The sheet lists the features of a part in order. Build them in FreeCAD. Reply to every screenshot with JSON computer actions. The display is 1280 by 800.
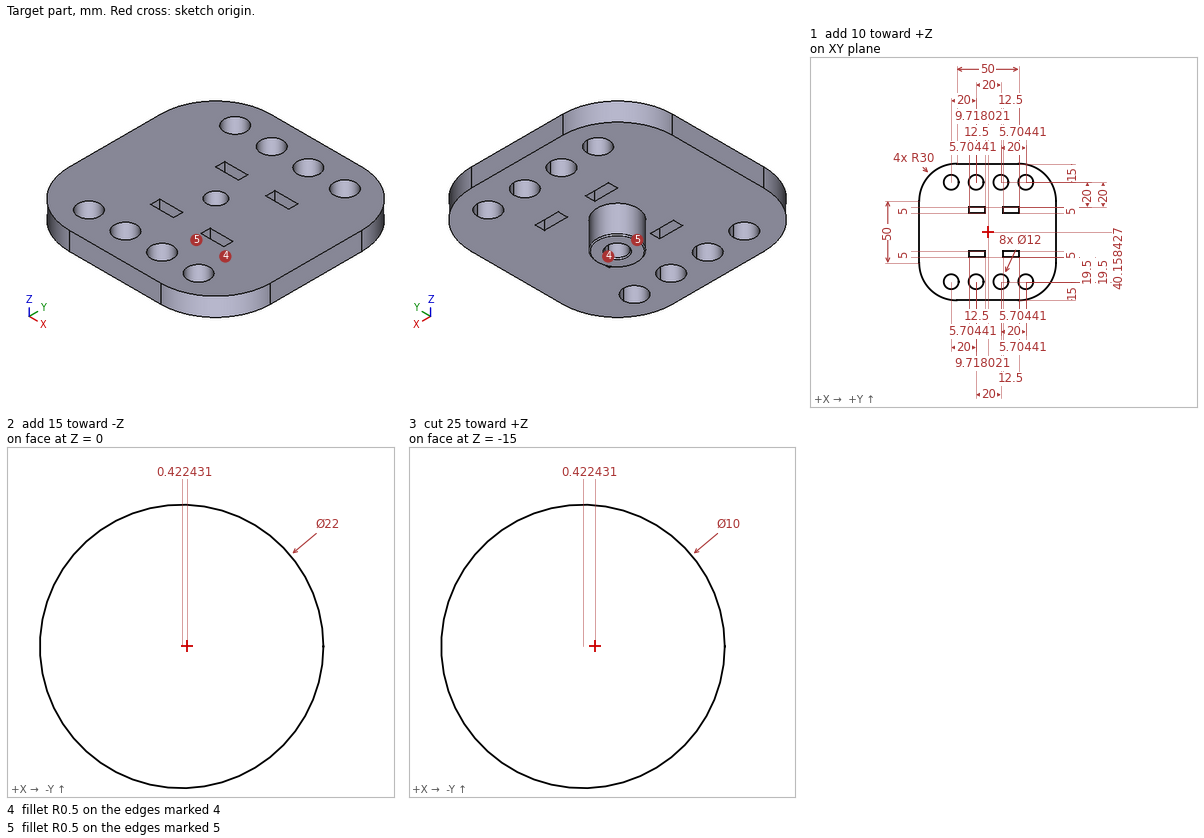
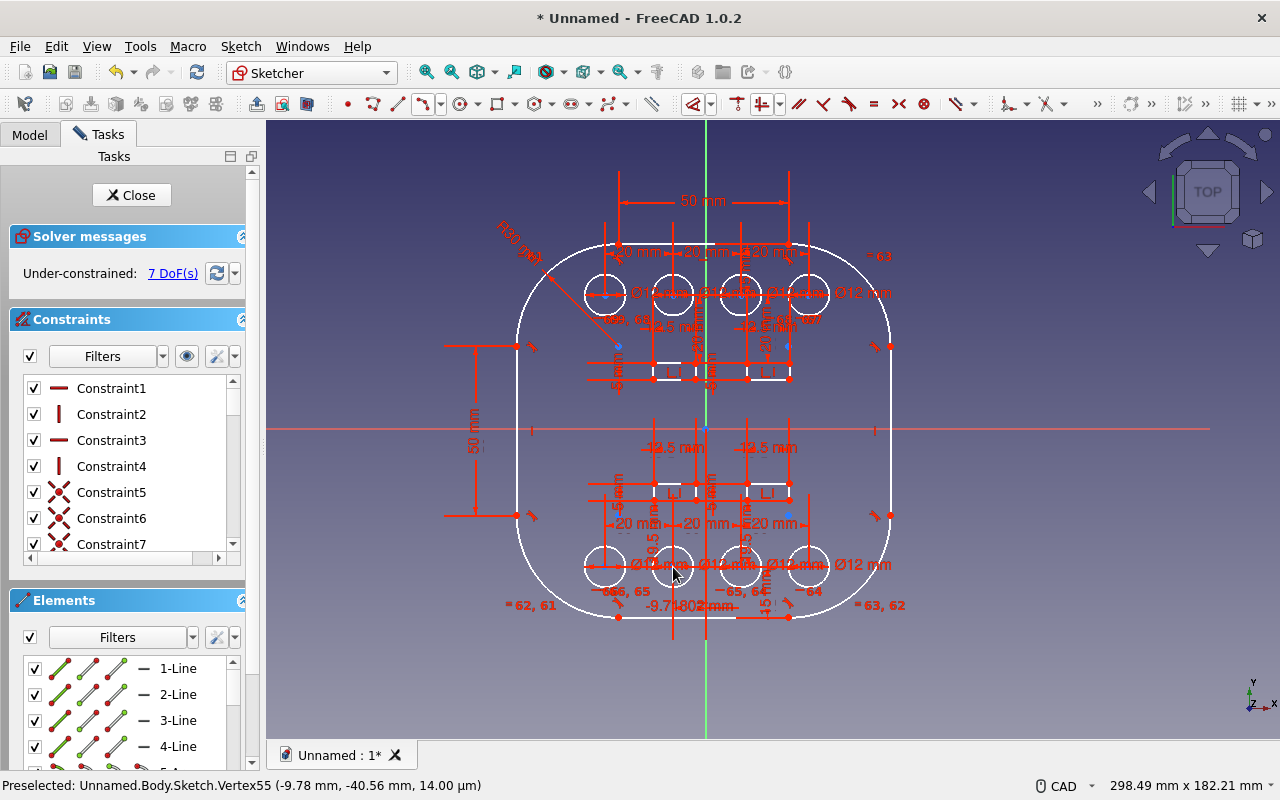
{"action": "left_click", "coordinate": [673, 295]}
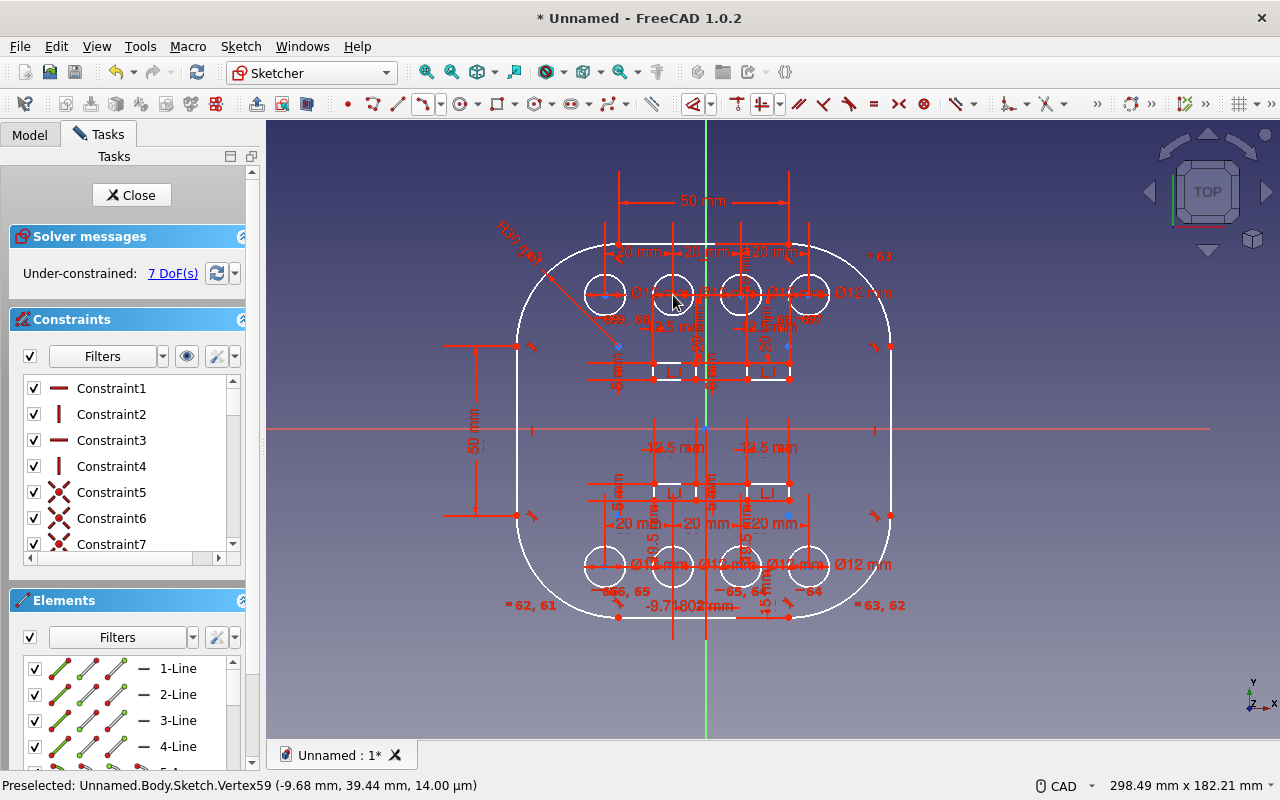
{"action": "key", "text": "l"}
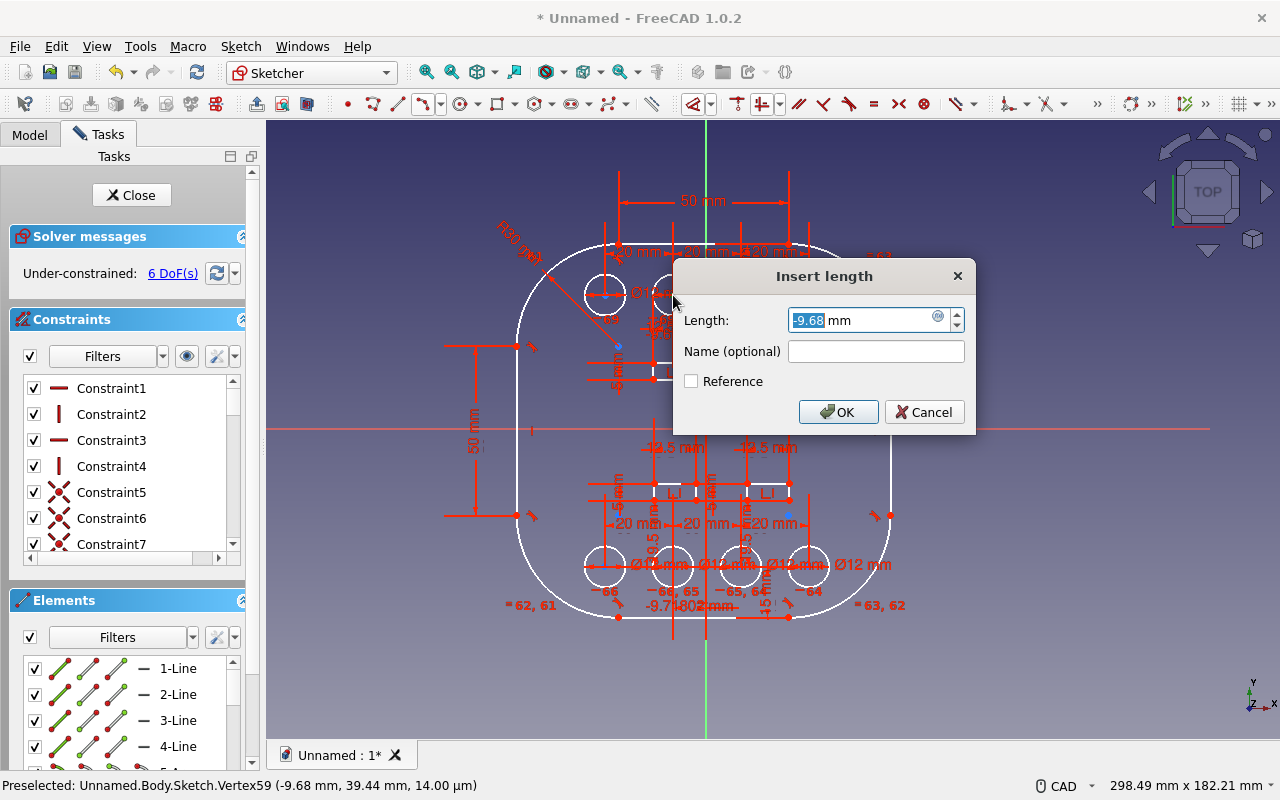
{"action": "type", "text": "-9.718021"}
{"action": "key", "text": "Return"}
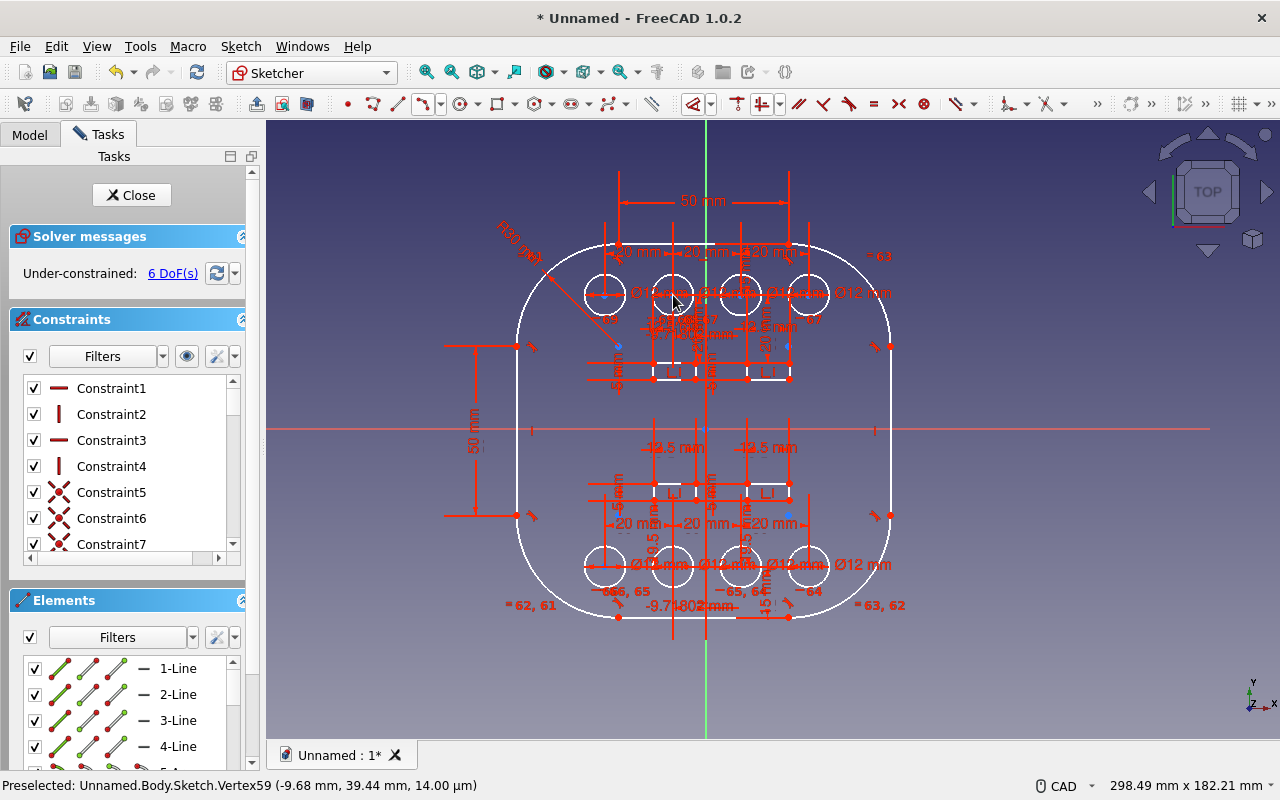
{"action": "scroll", "coordinate": [789, 618], "scroll_direction": "up", "scroll_amount": 4}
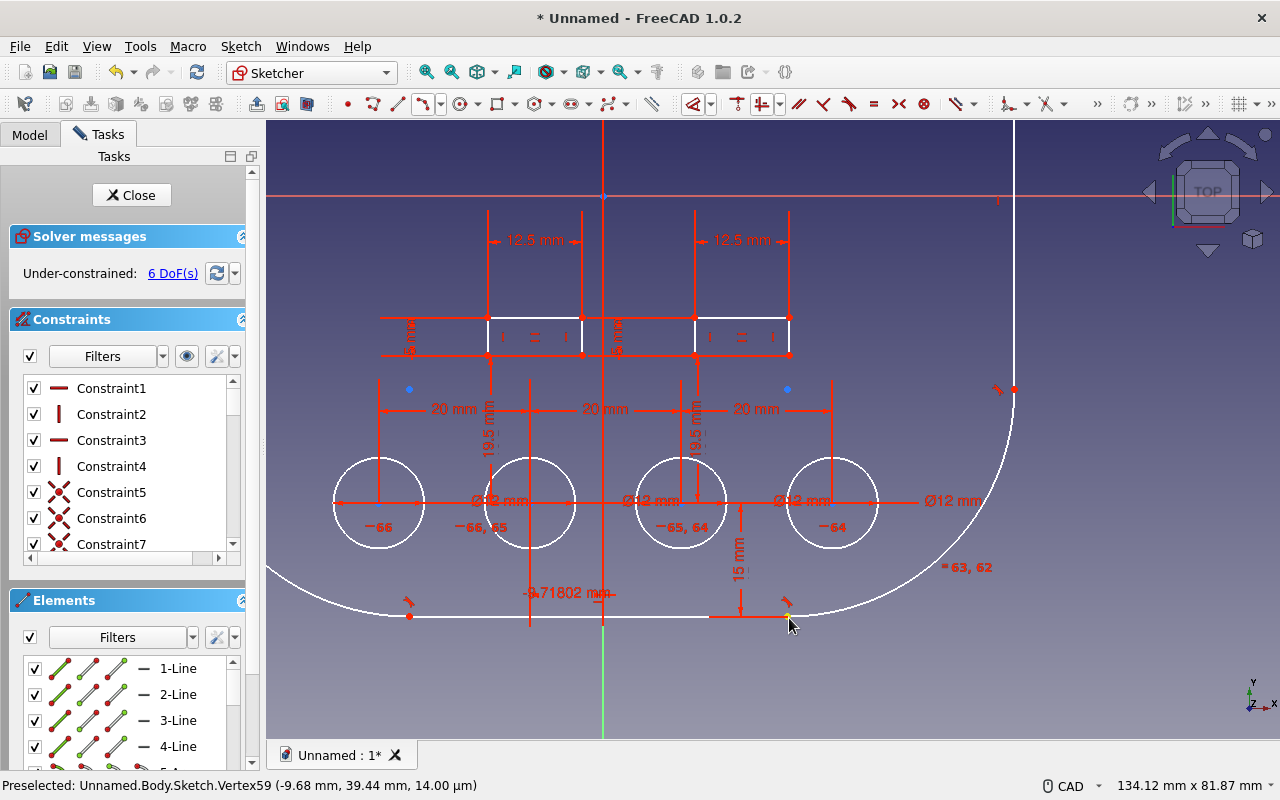
{"action": "left_click", "coordinate": [787, 617]}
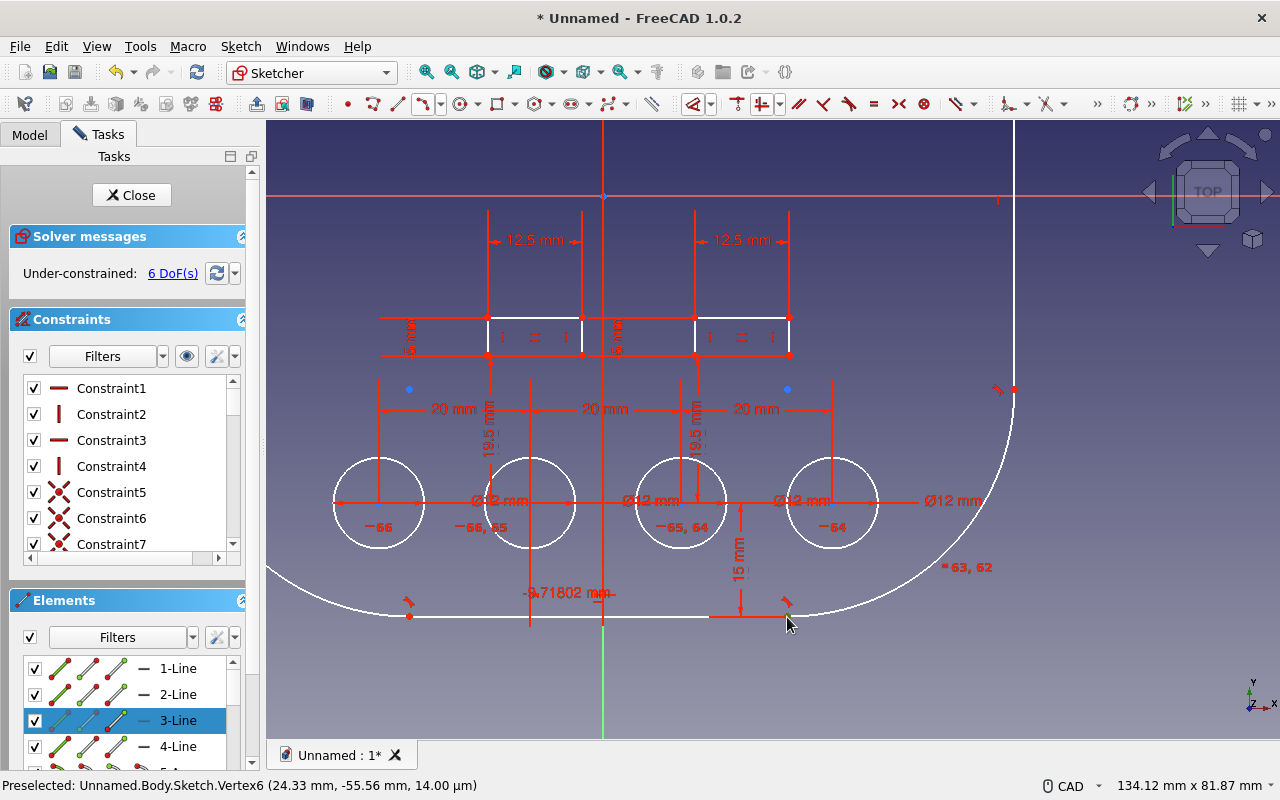
{"action": "left_click", "coordinate": [832, 503]}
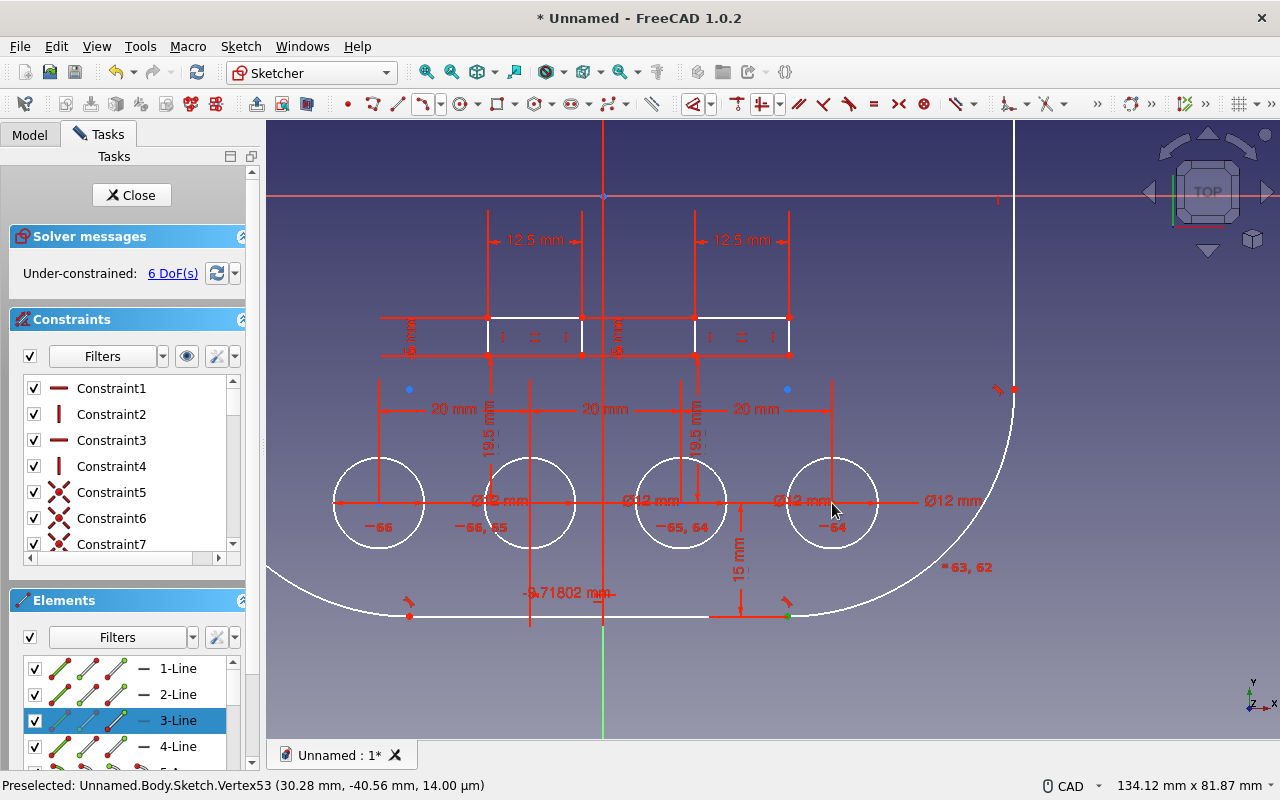
{"action": "key", "text": "l"}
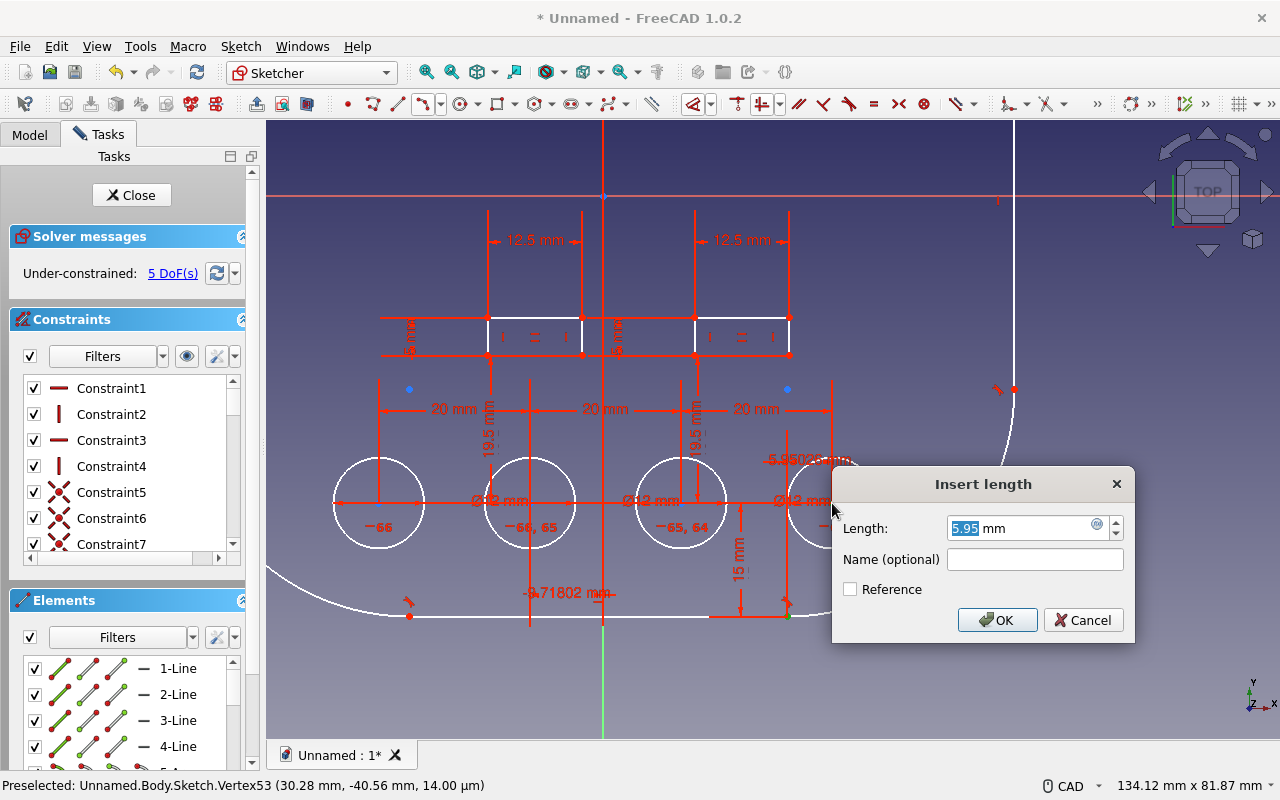
{"action": "type", "text": "5.70441"}
{"action": "key", "text": "Return"}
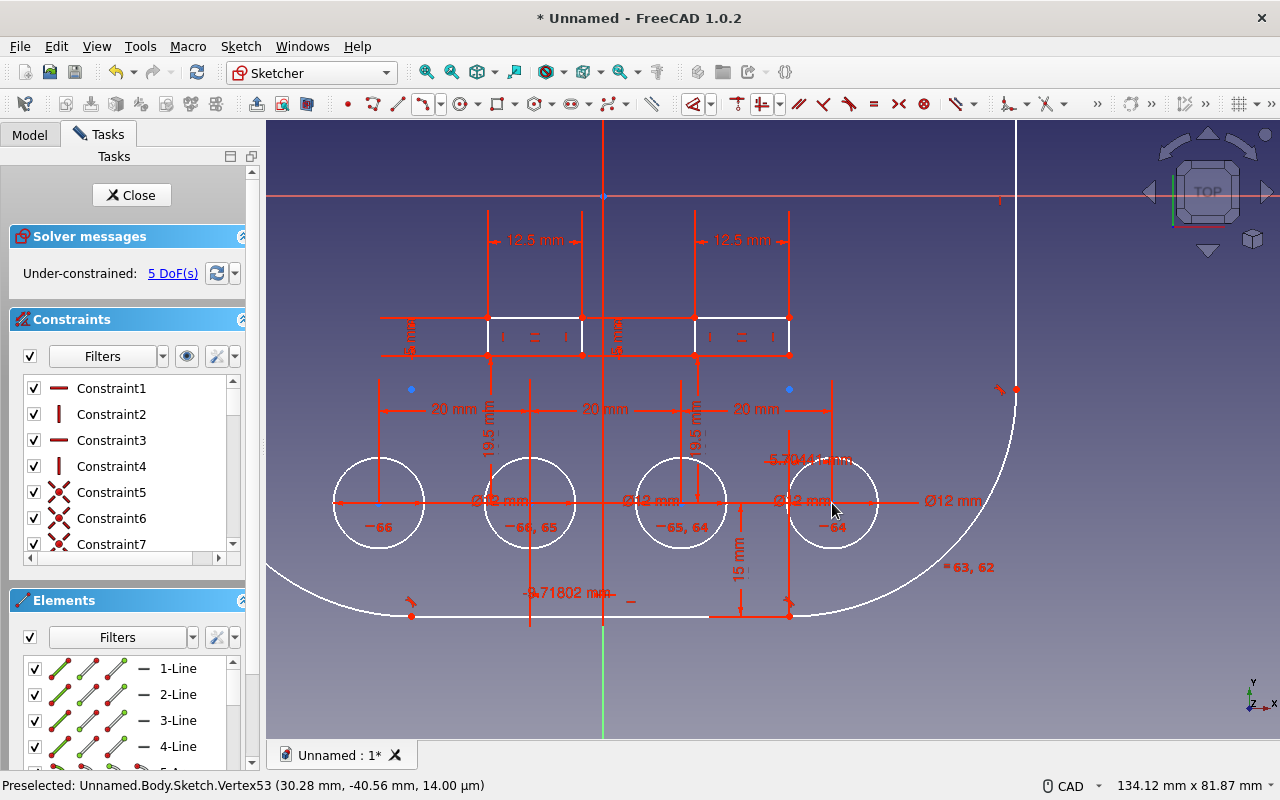
{"action": "left_click", "coordinate": [789, 356]}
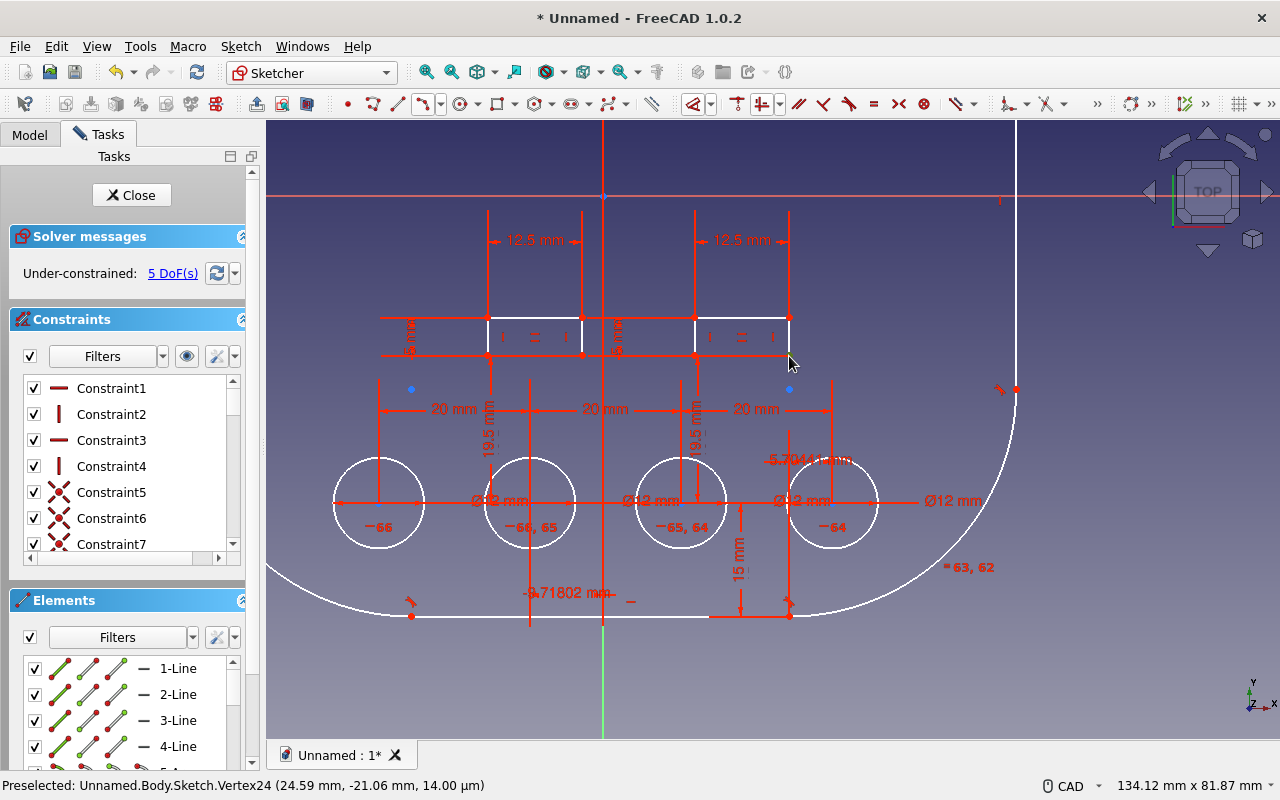
{"action": "left_click", "coordinate": [832, 503]}